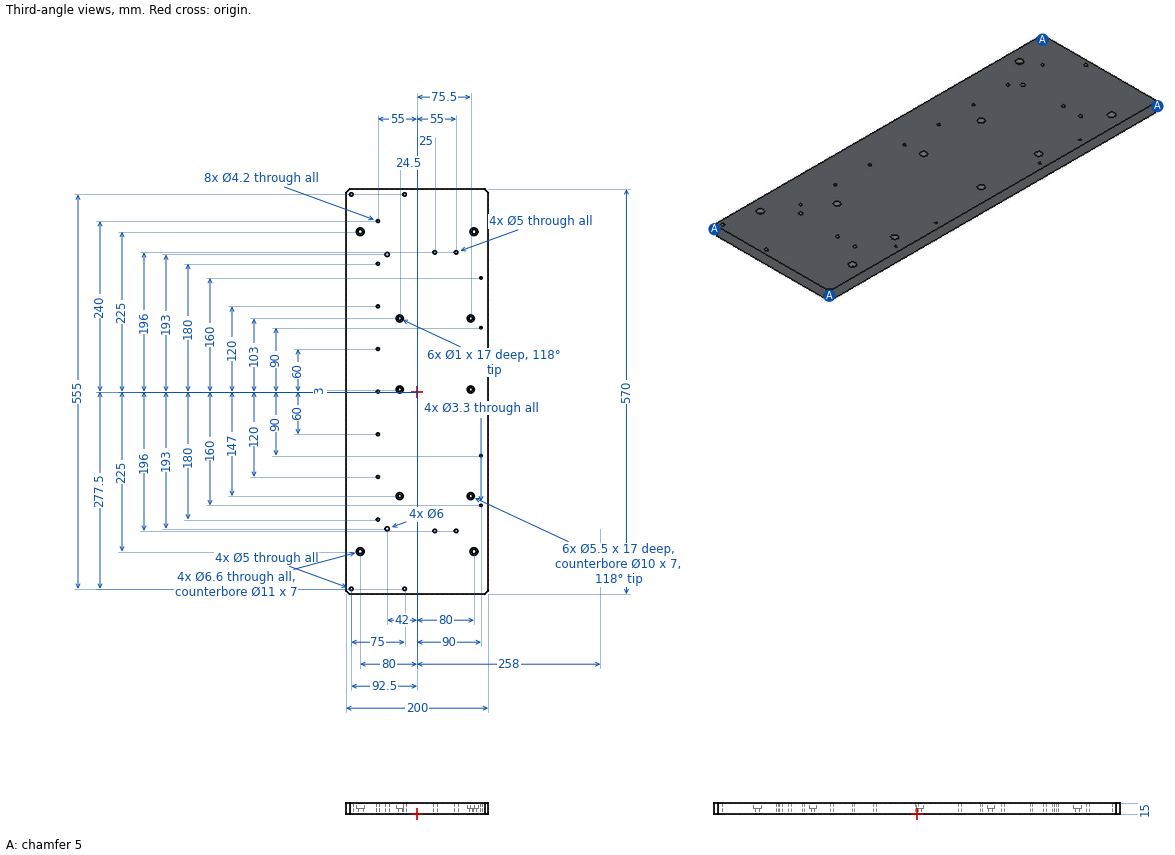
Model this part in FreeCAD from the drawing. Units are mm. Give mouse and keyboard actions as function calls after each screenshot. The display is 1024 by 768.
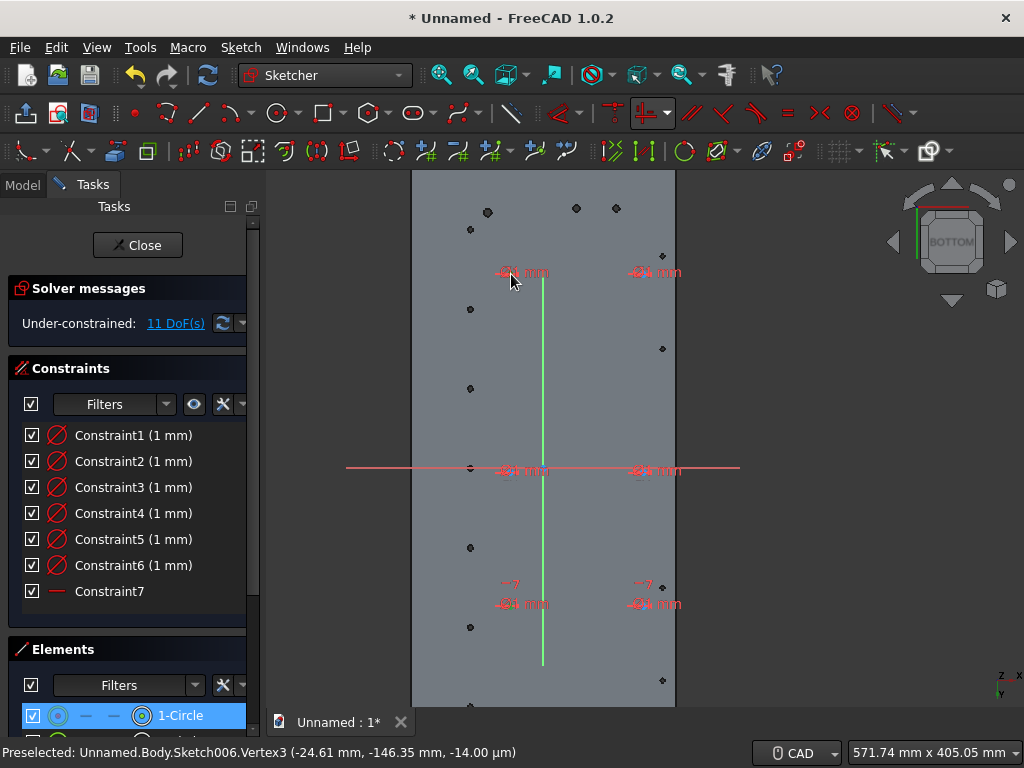
key(v)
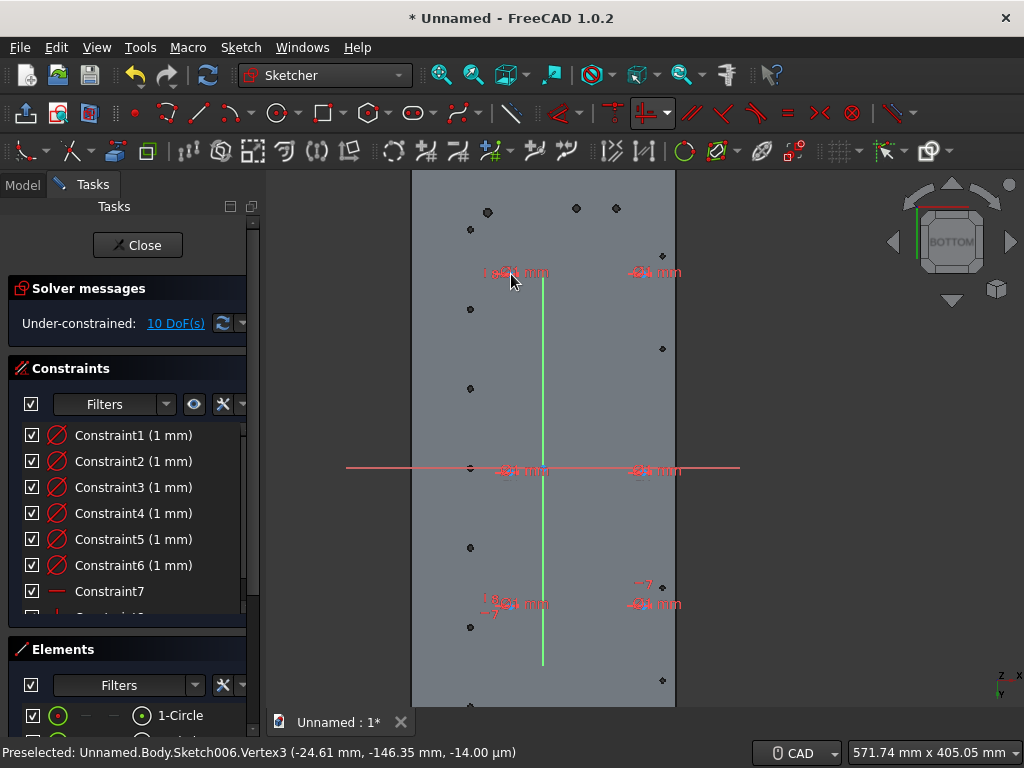
click(643, 606)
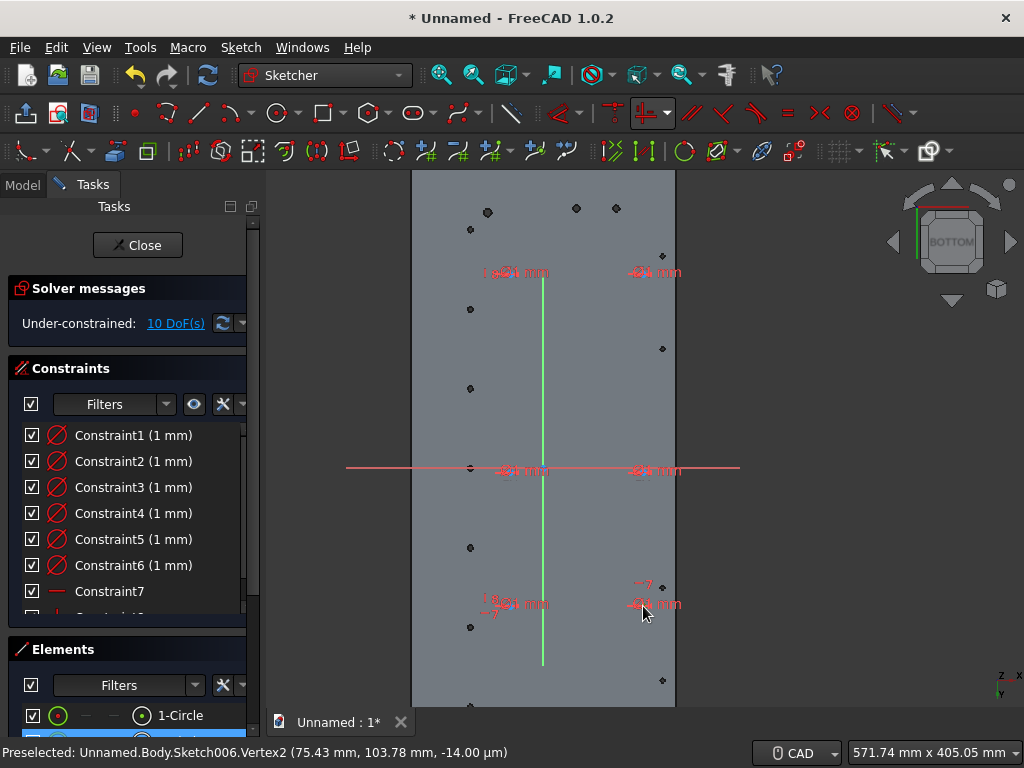
click(643, 274)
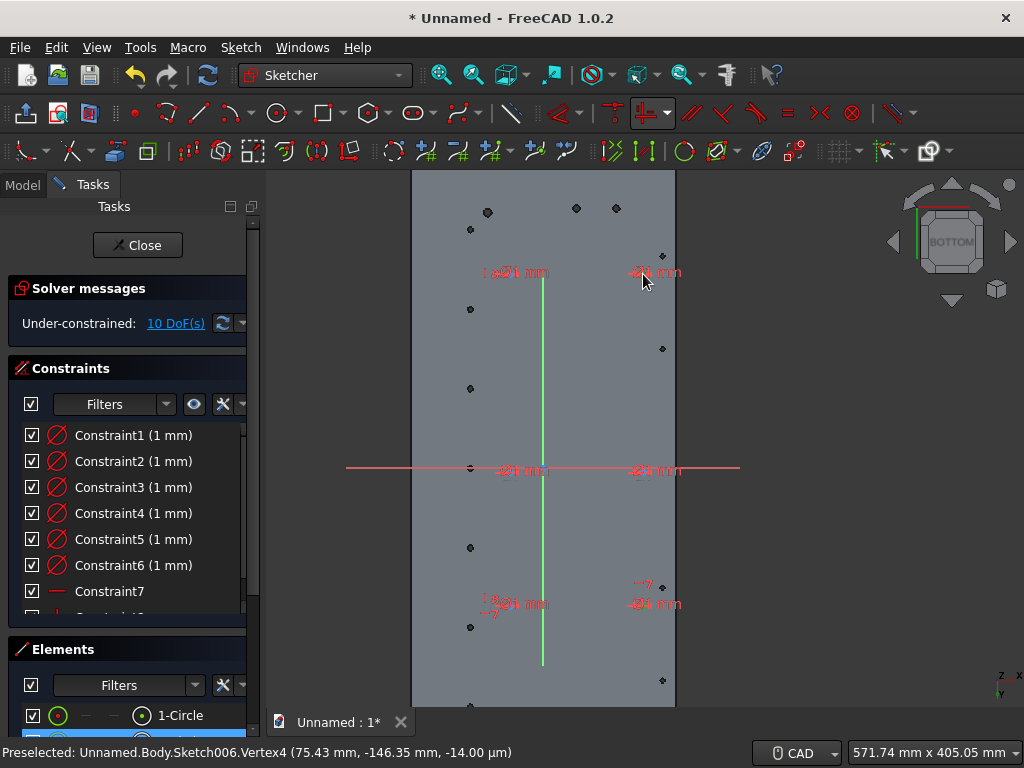
click(670, 114)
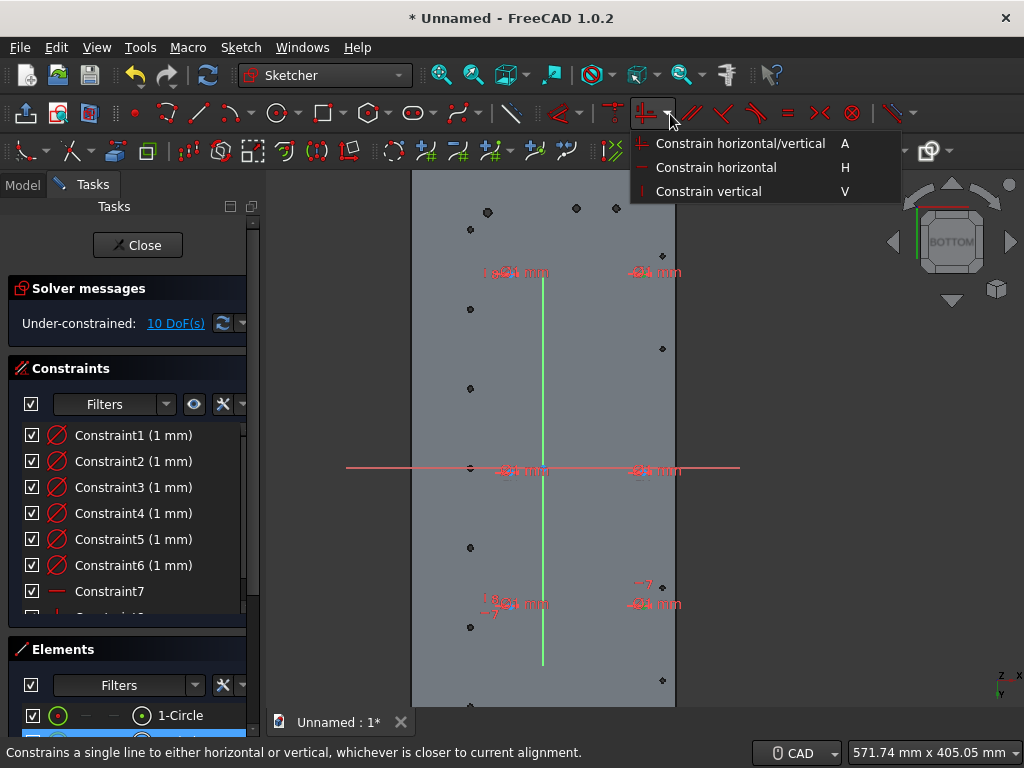
click(766, 191)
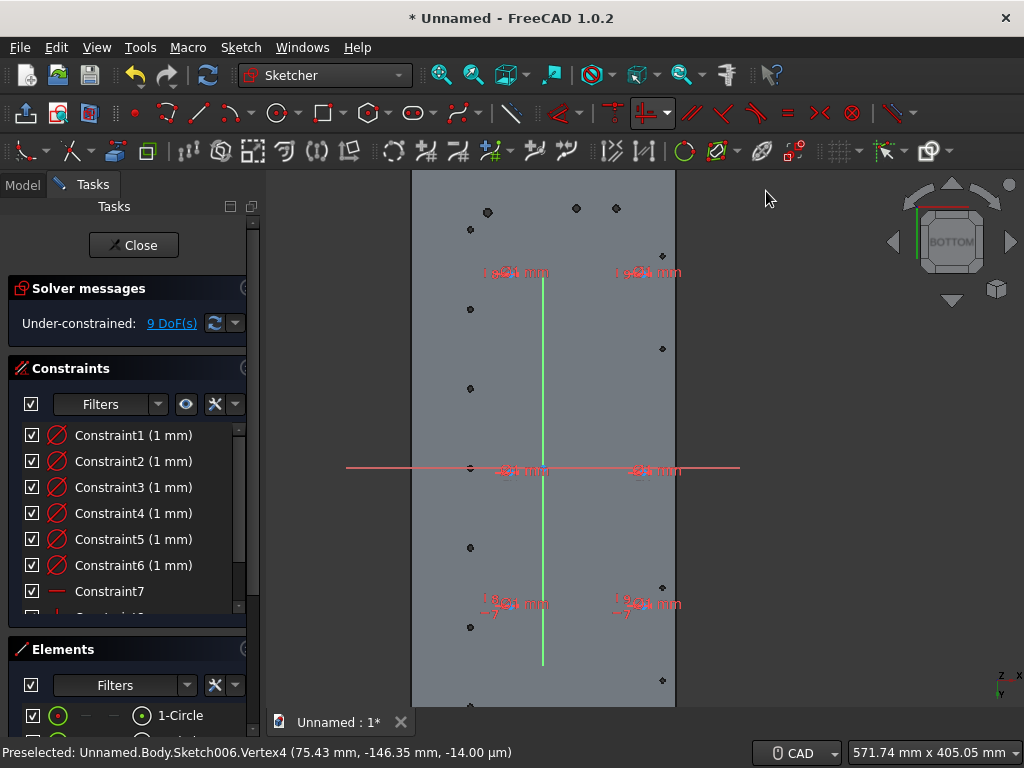
click(511, 274)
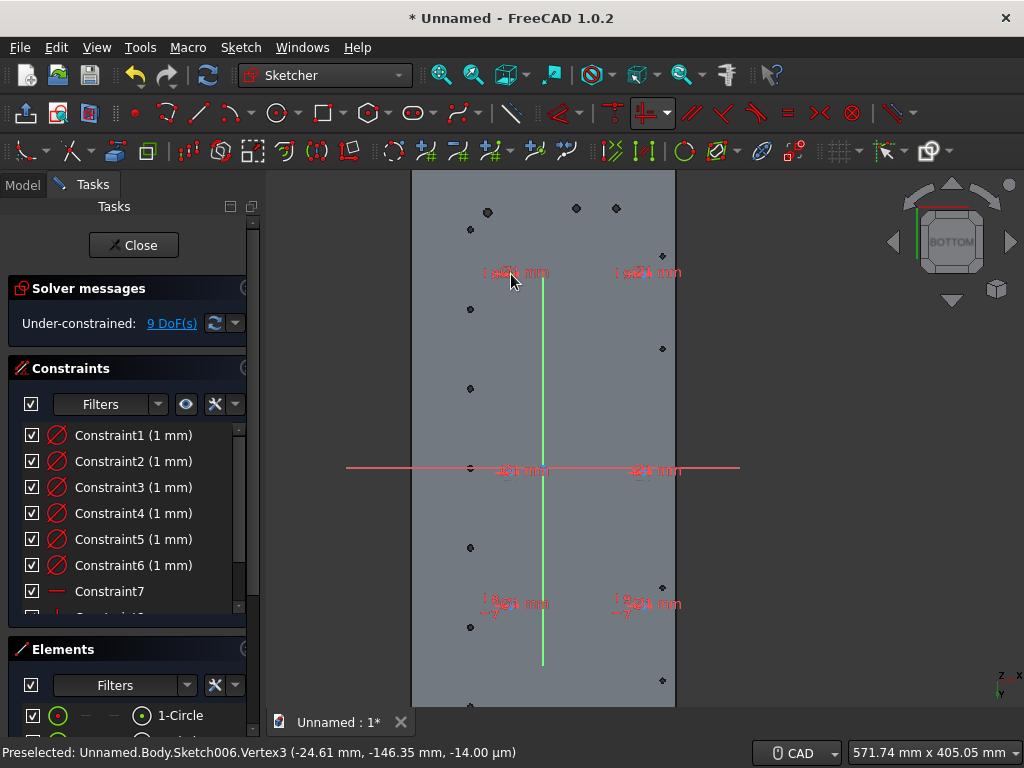
click(643, 274)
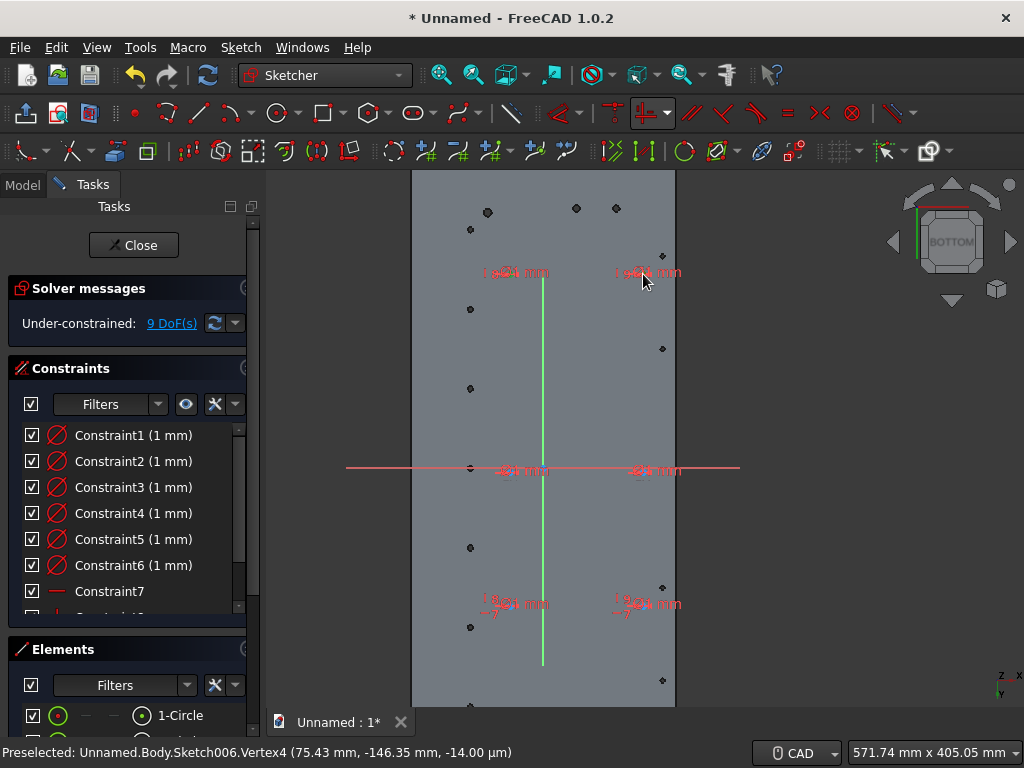
click(670, 114)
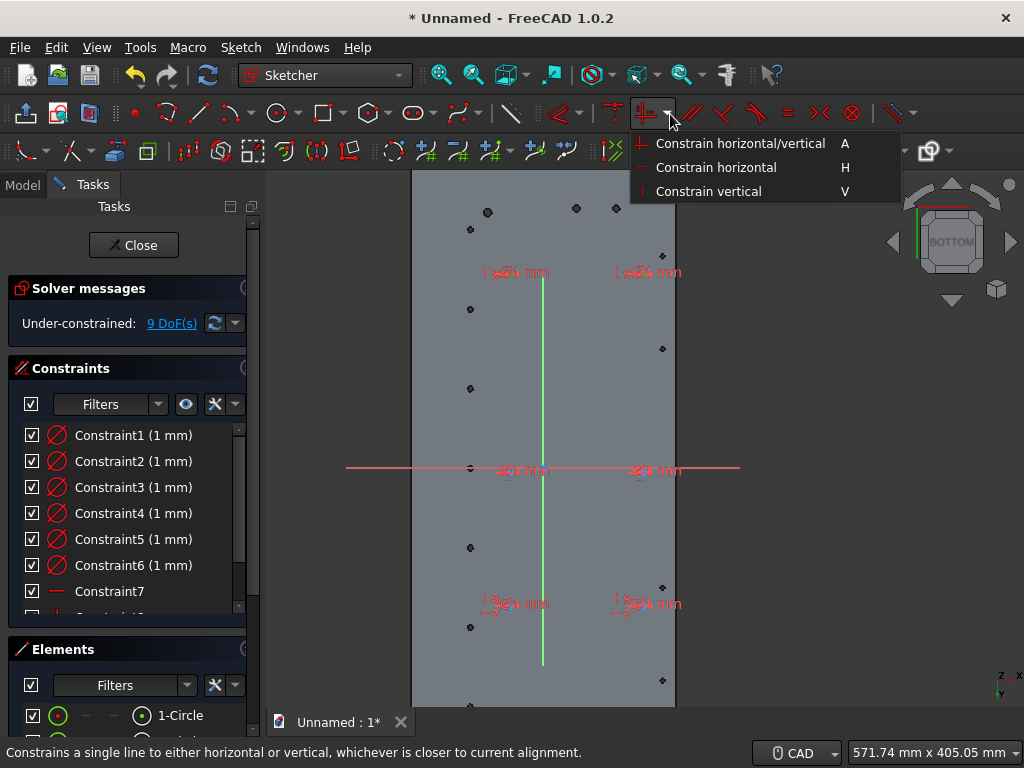
click(766, 167)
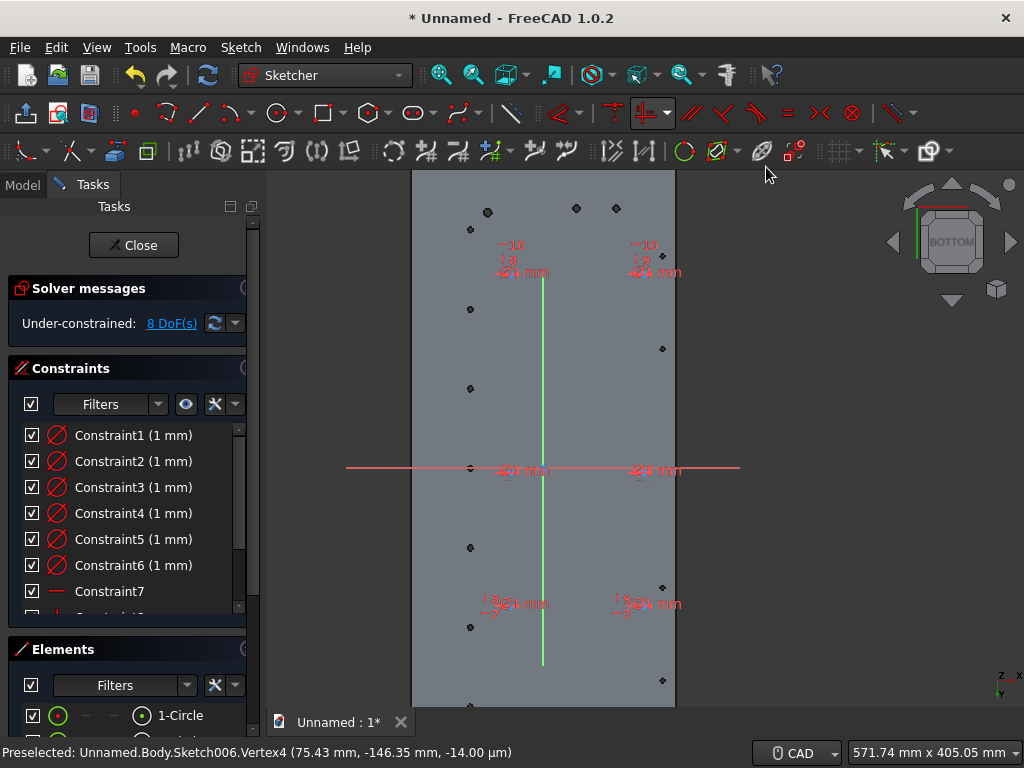
click(511, 606)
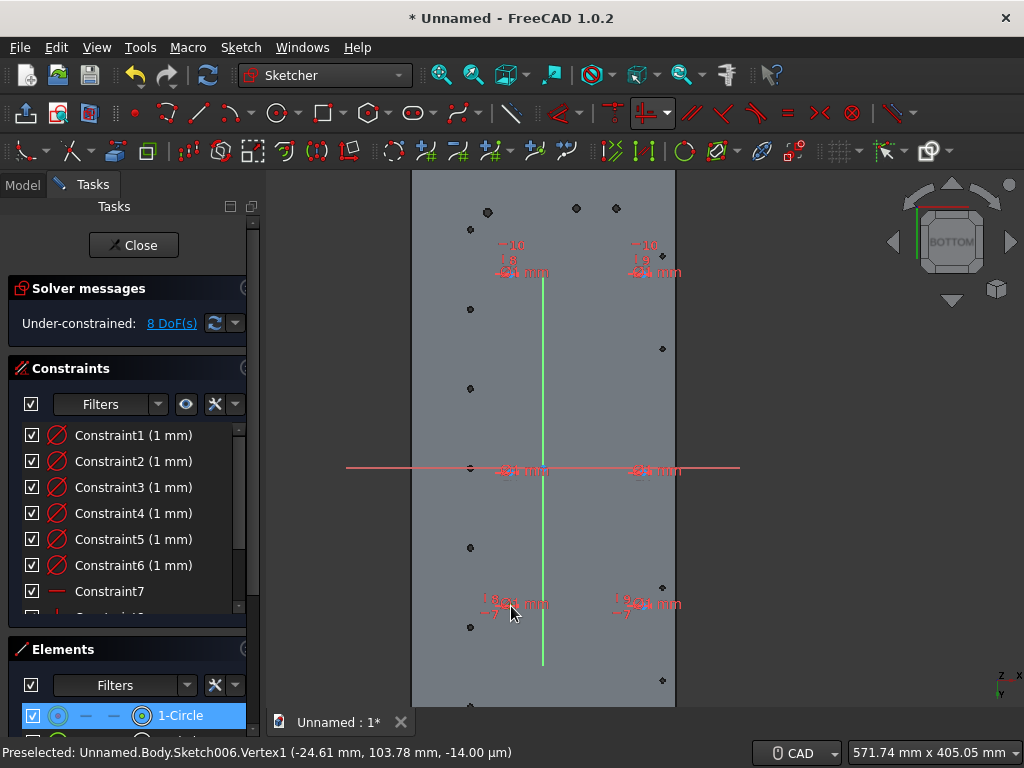
click(511, 473)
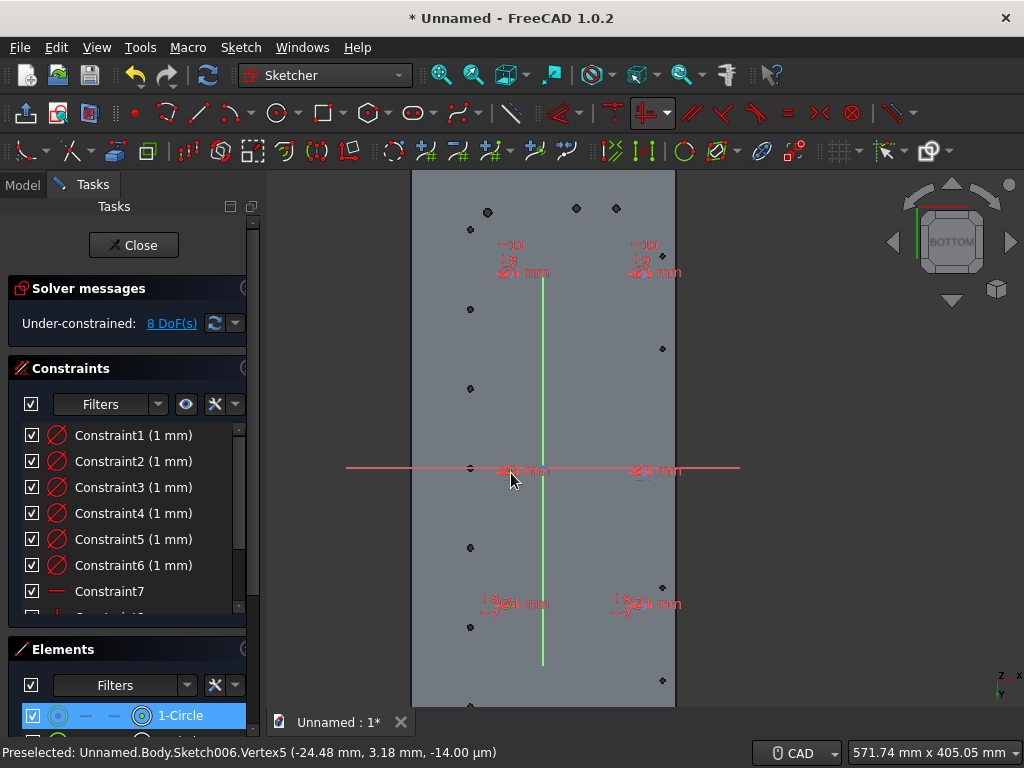
click(670, 114)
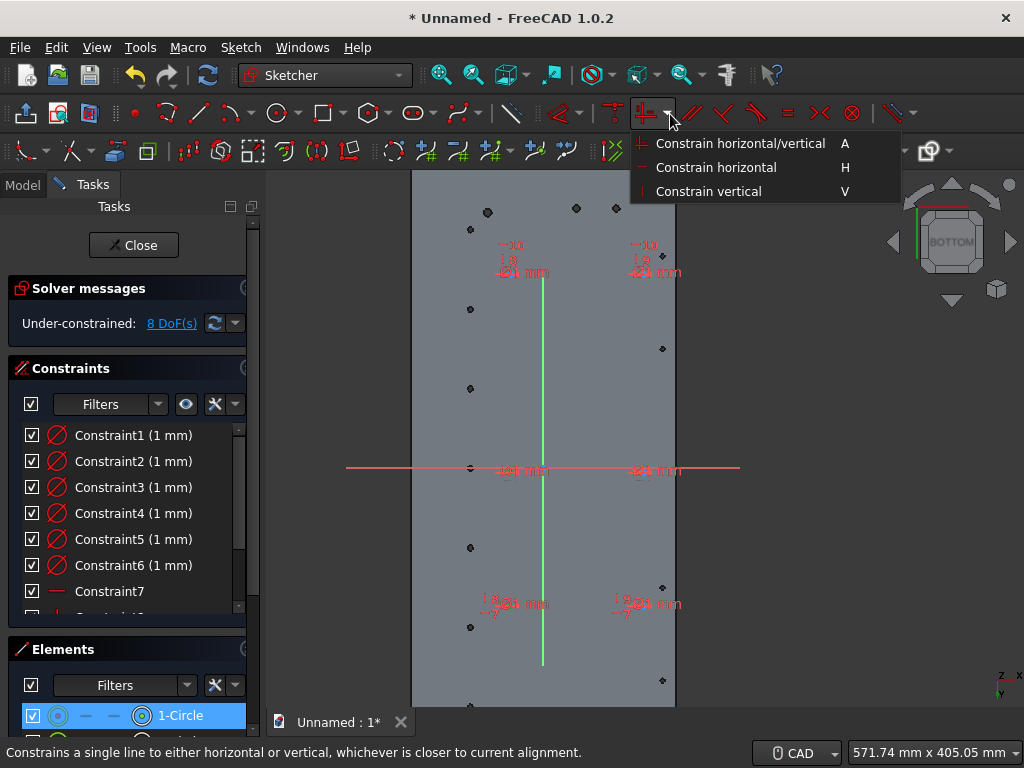
click(766, 191)